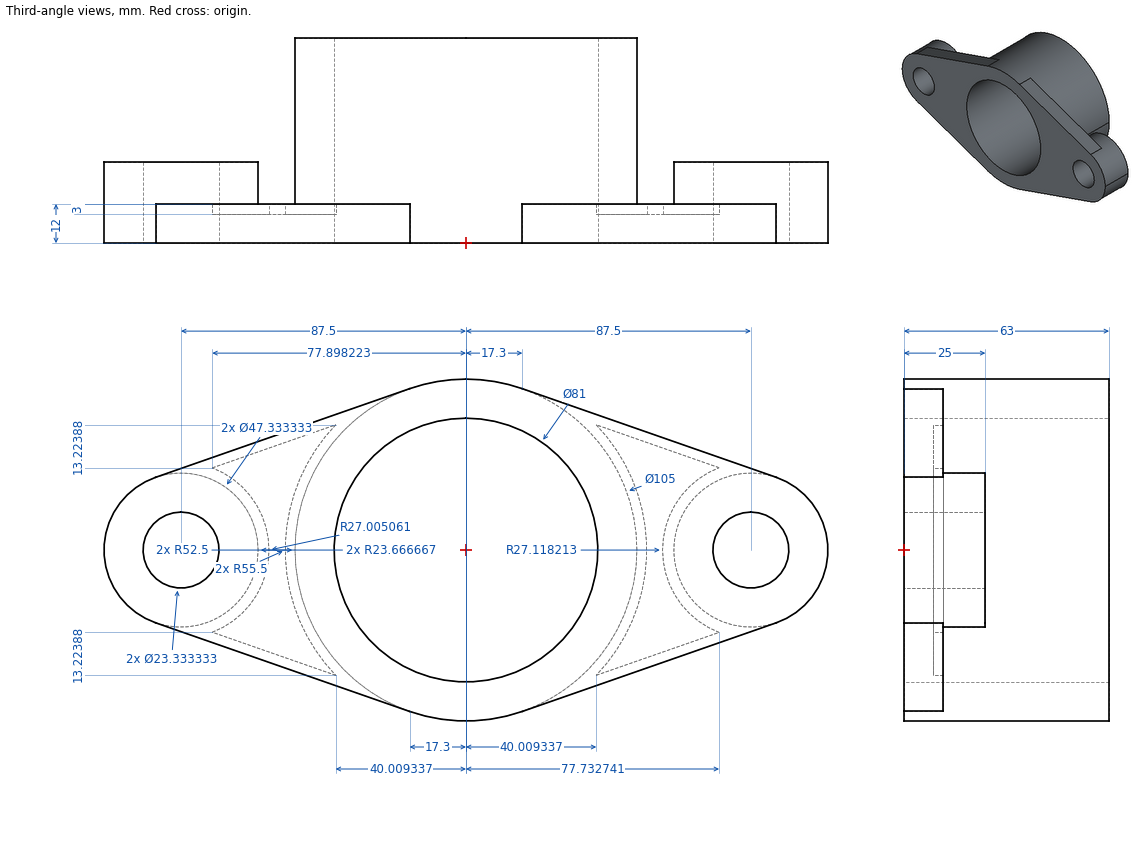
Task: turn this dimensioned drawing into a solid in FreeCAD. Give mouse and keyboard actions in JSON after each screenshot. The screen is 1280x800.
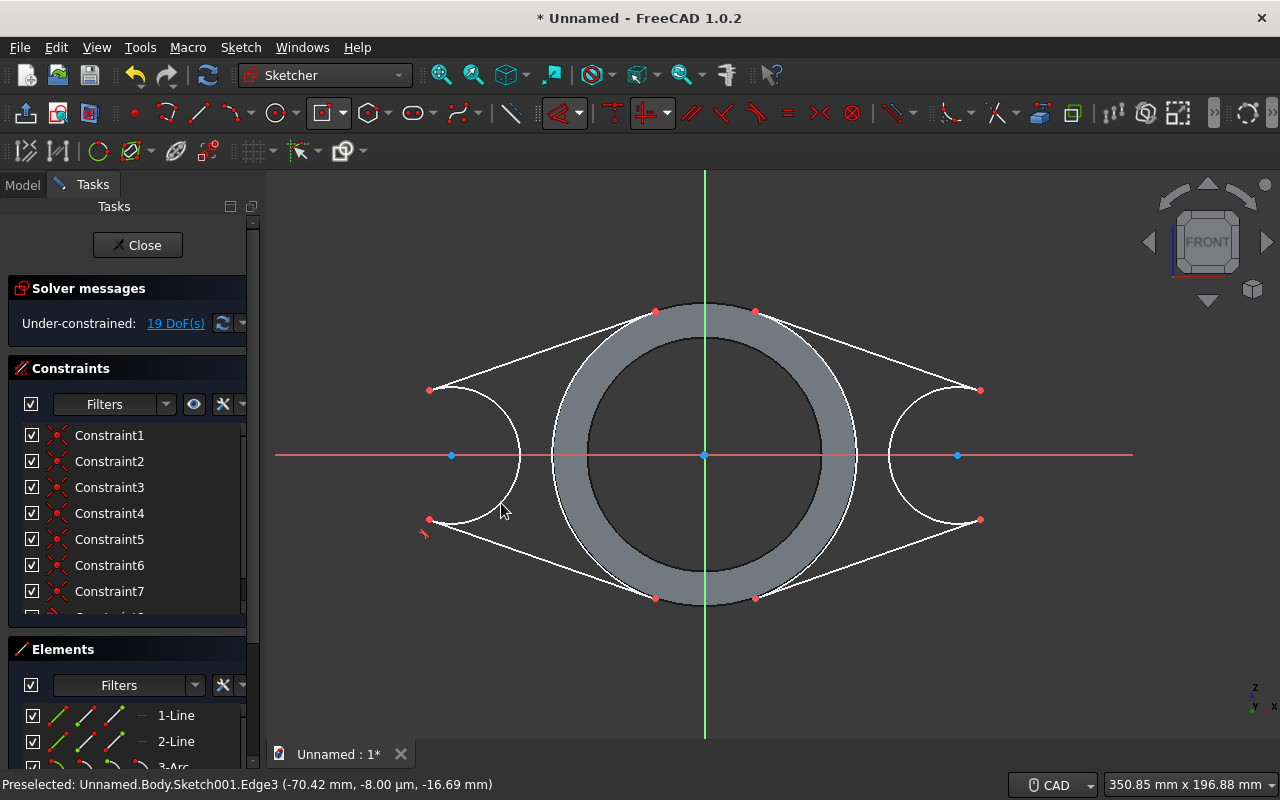
{"action": "left_click", "coordinate": [497, 367]}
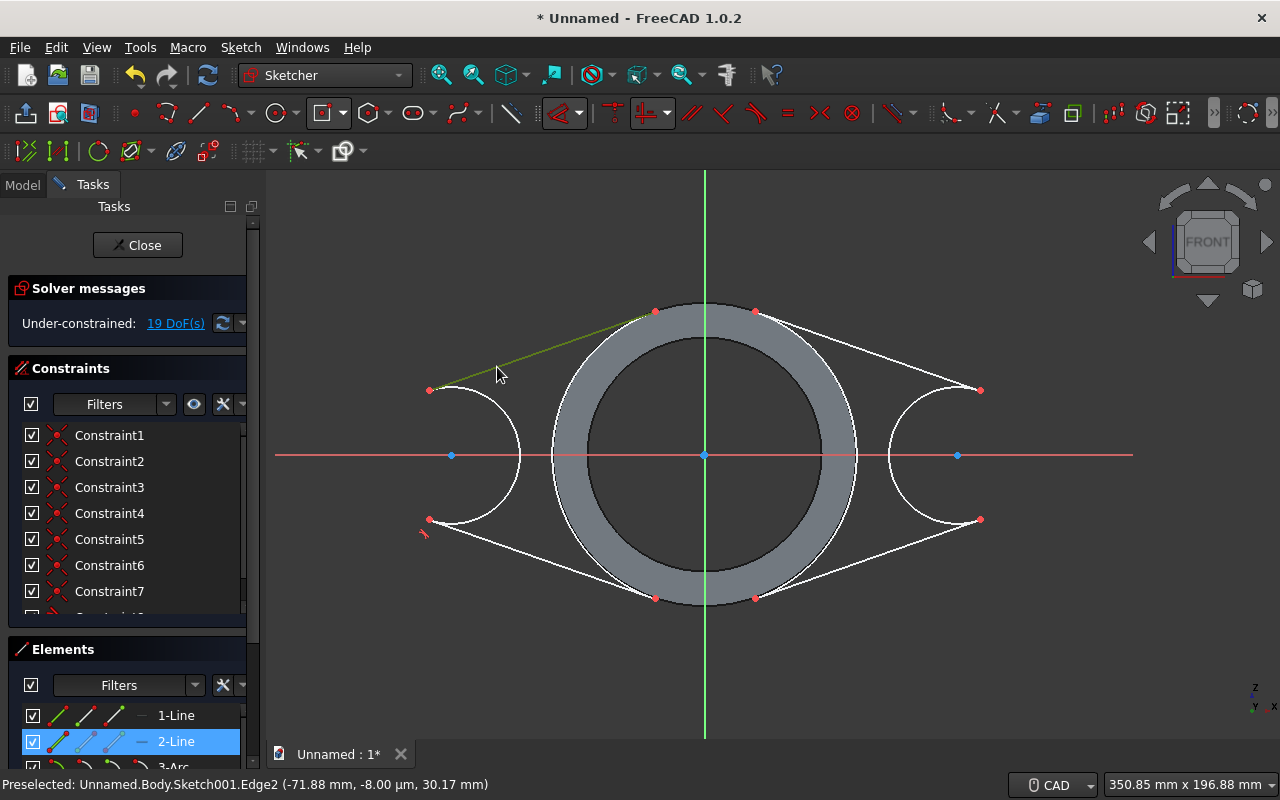
{"action": "left_click", "coordinate": [501, 503]}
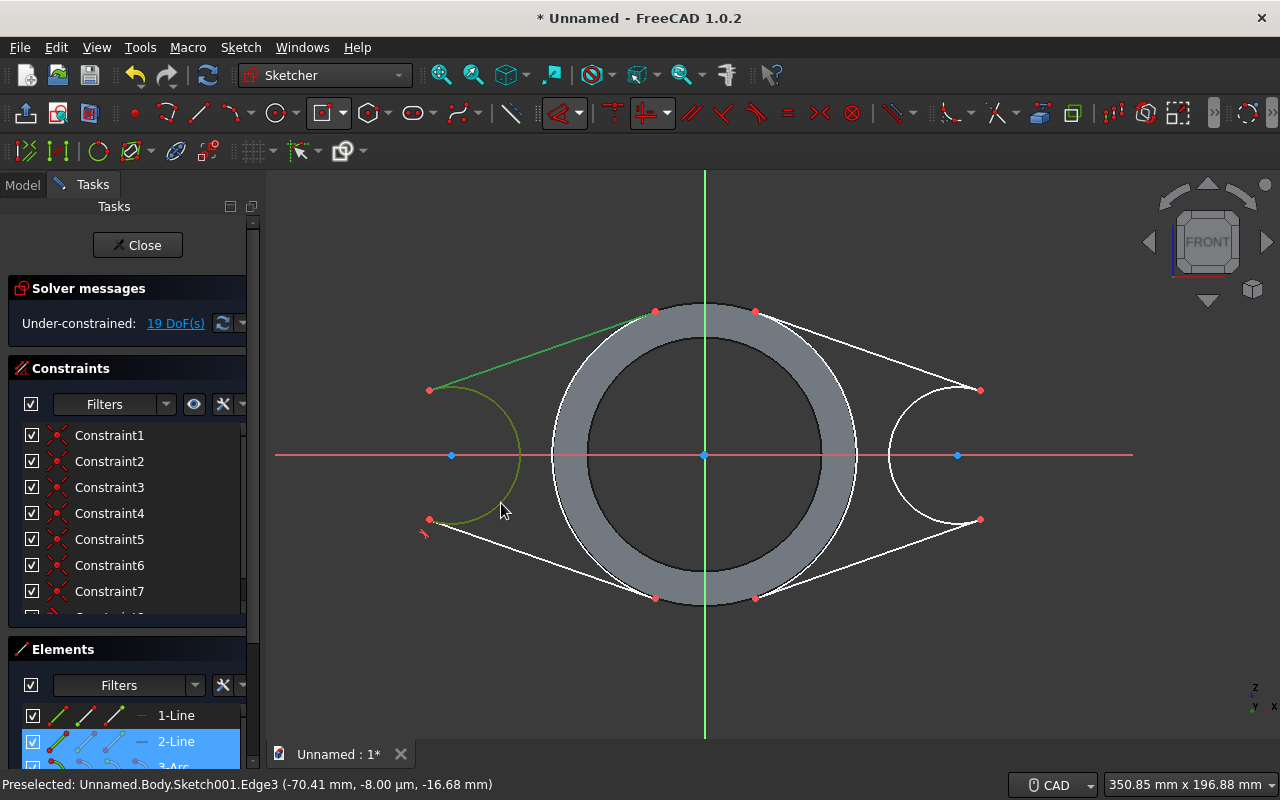
{"action": "key", "text": "t"}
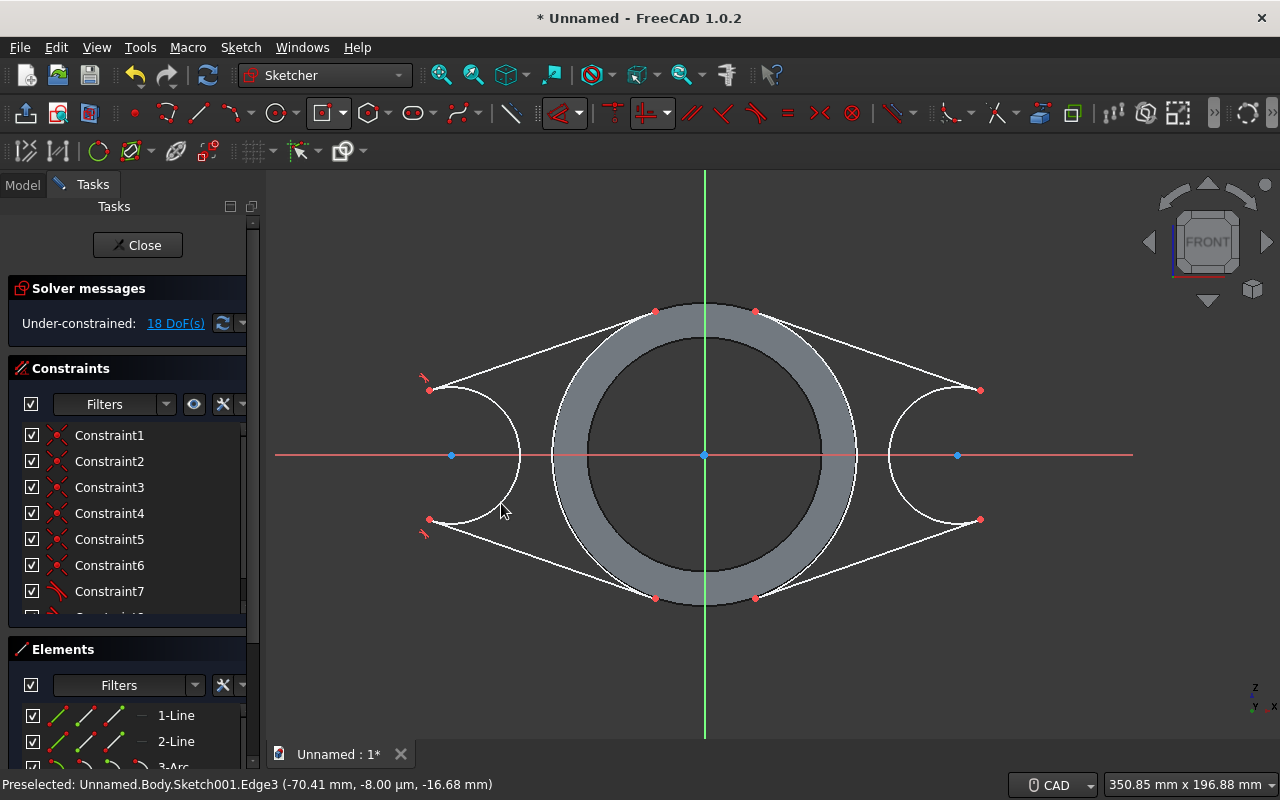
{"action": "left_click", "coordinate": [913, 544]}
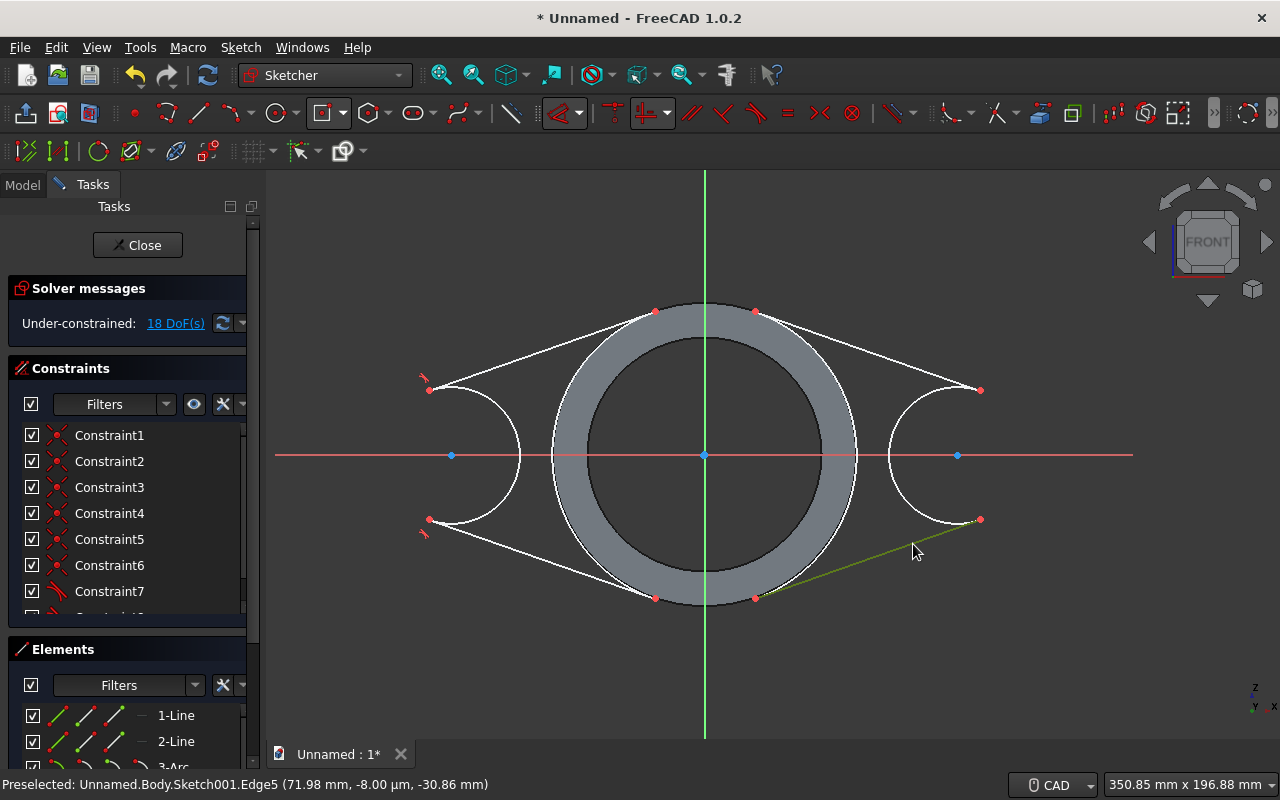
{"action": "left_click", "coordinate": [839, 528]}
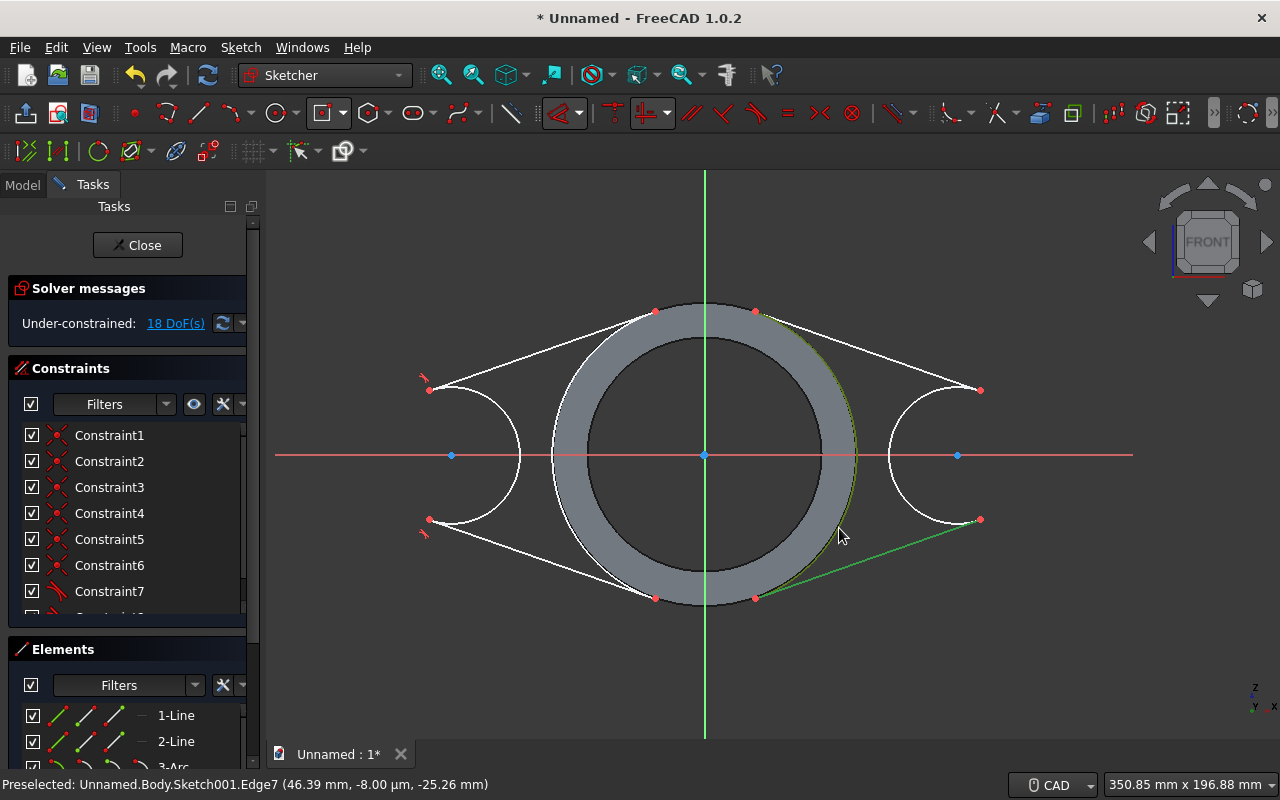
{"action": "key", "text": "t"}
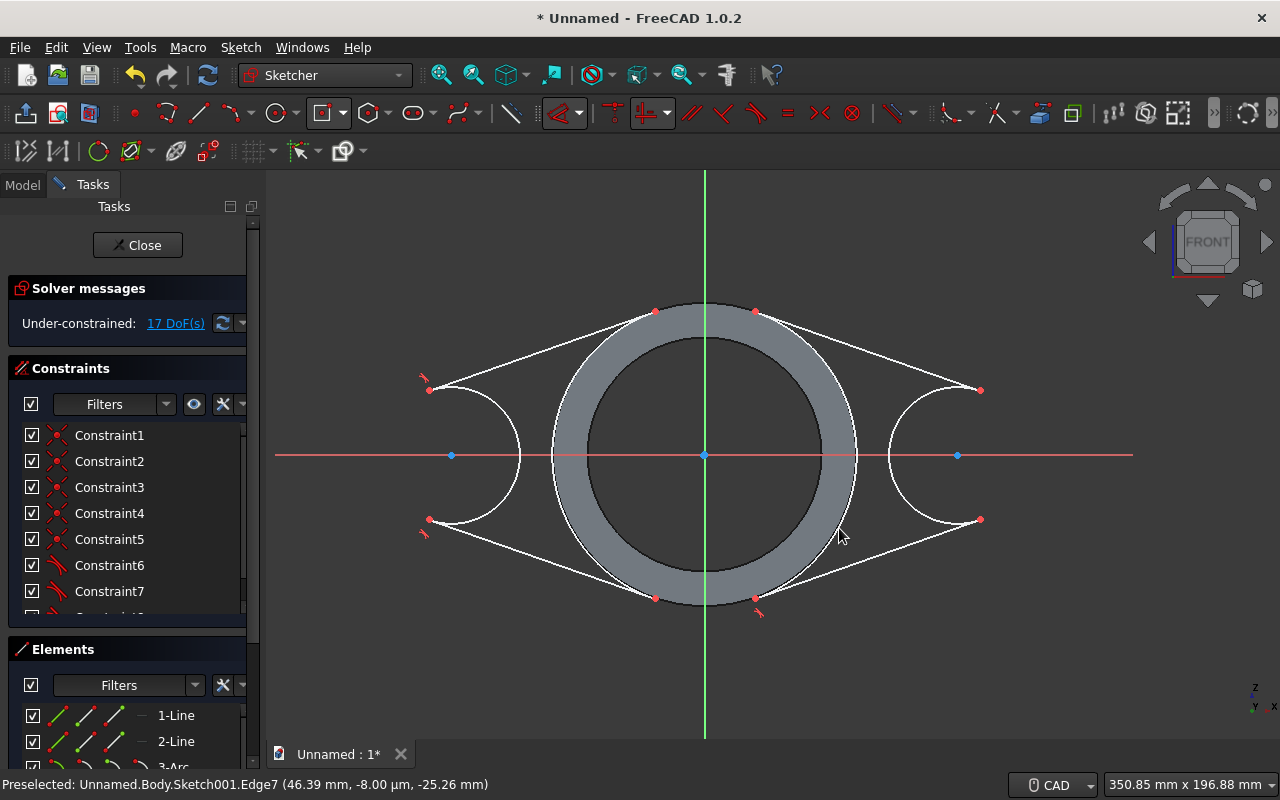
{"action": "left_click", "coordinate": [913, 544]}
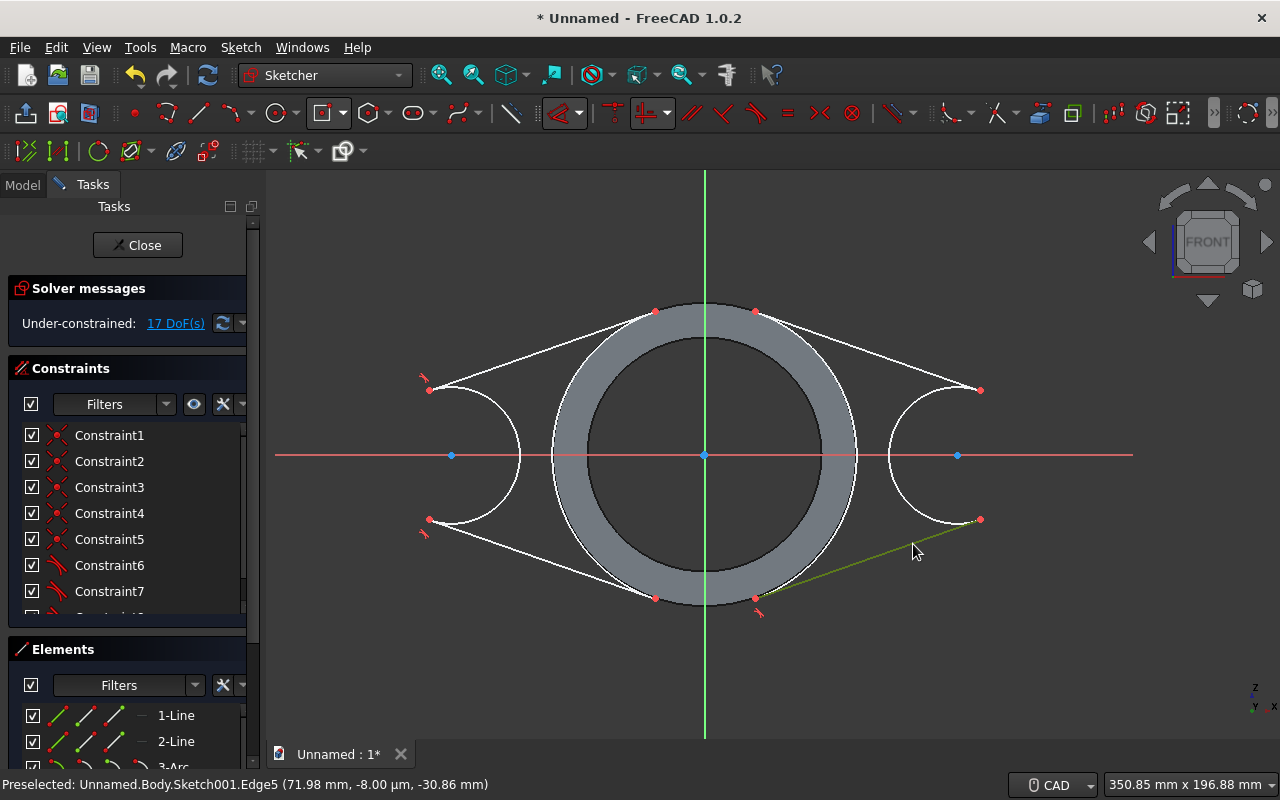
{"action": "left_click", "coordinate": [908, 408]}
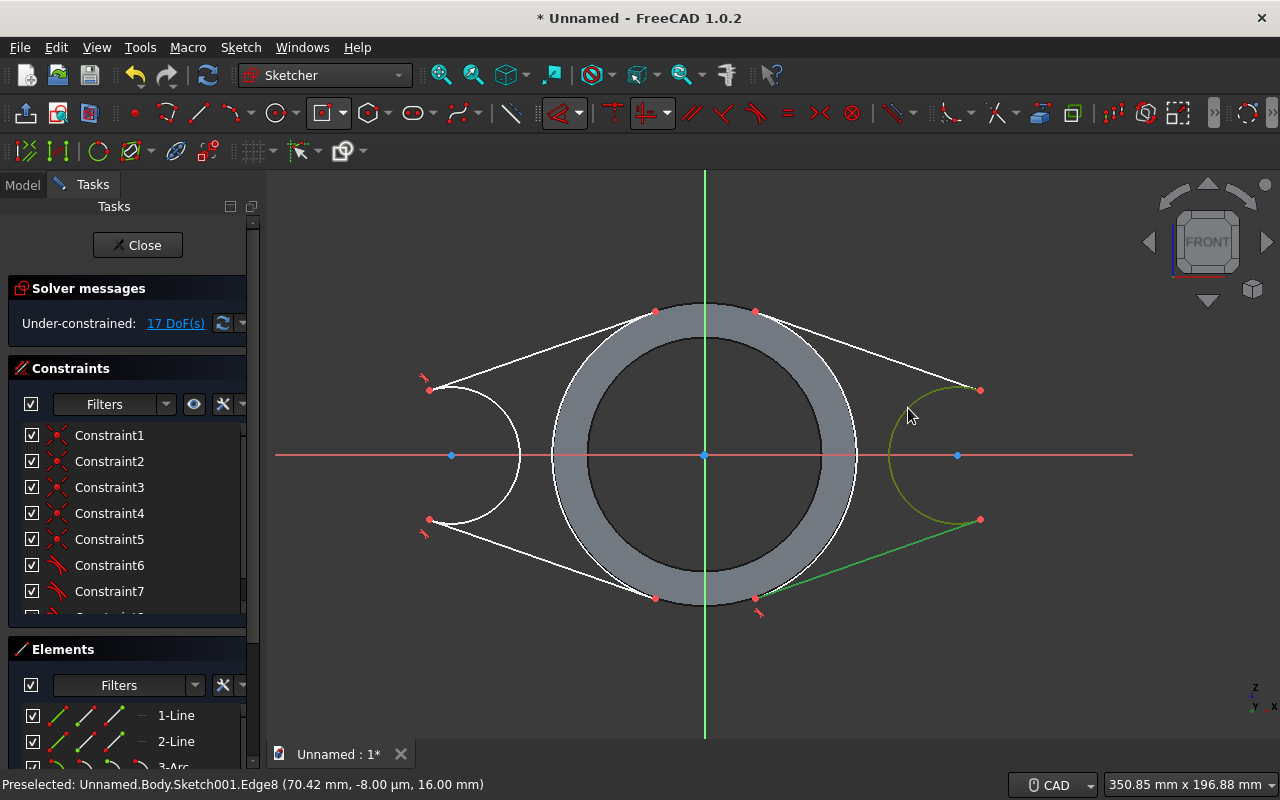
{"action": "key", "text": "t"}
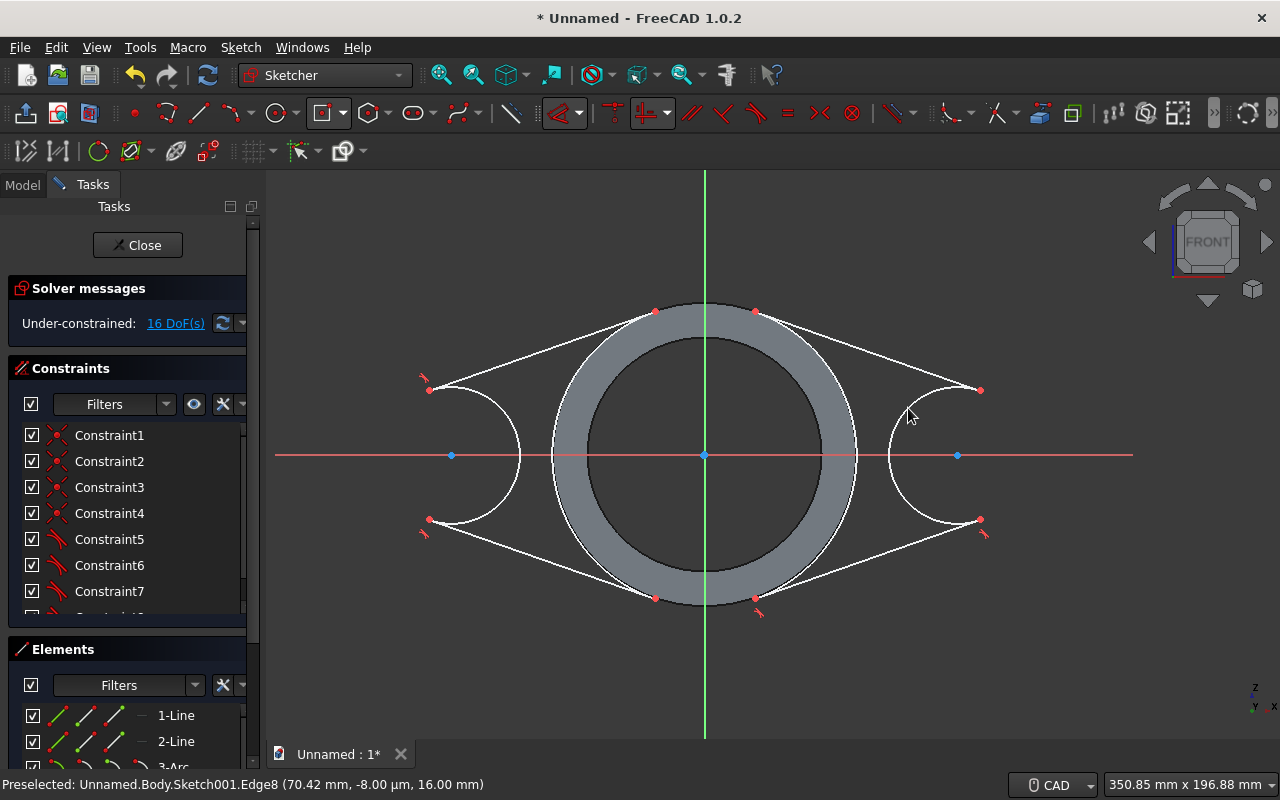
{"action": "left_click", "coordinate": [823, 336]}